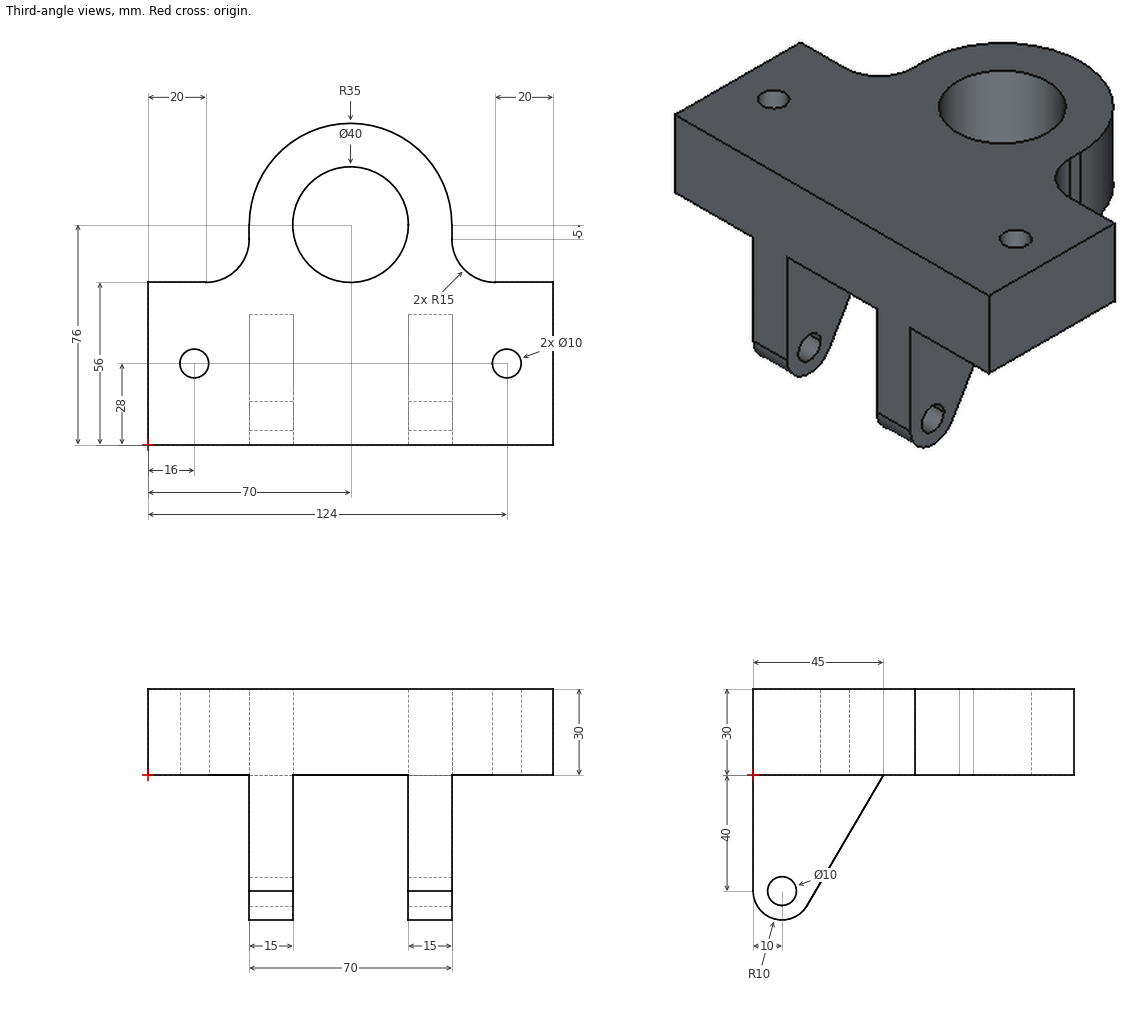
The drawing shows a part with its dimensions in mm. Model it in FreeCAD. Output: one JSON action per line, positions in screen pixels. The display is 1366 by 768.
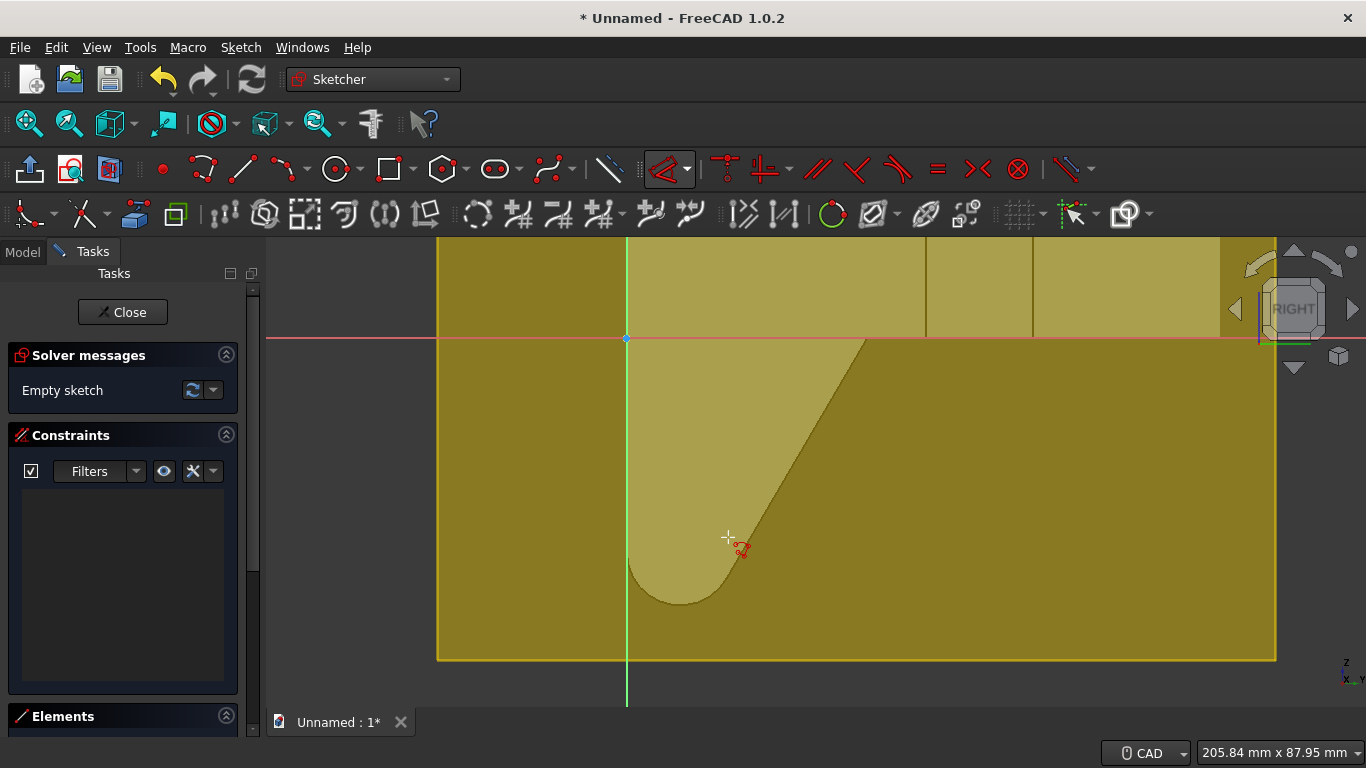
{"action": "left_click", "coordinate": [726, 579]}
{"action": "left_click", "coordinate": [867, 338]}
{"action": "left_click", "coordinate": [627, 338]}
{"action": "left_click", "coordinate": [636, 552]}
{"action": "right_click", "coordinate": [636, 552]}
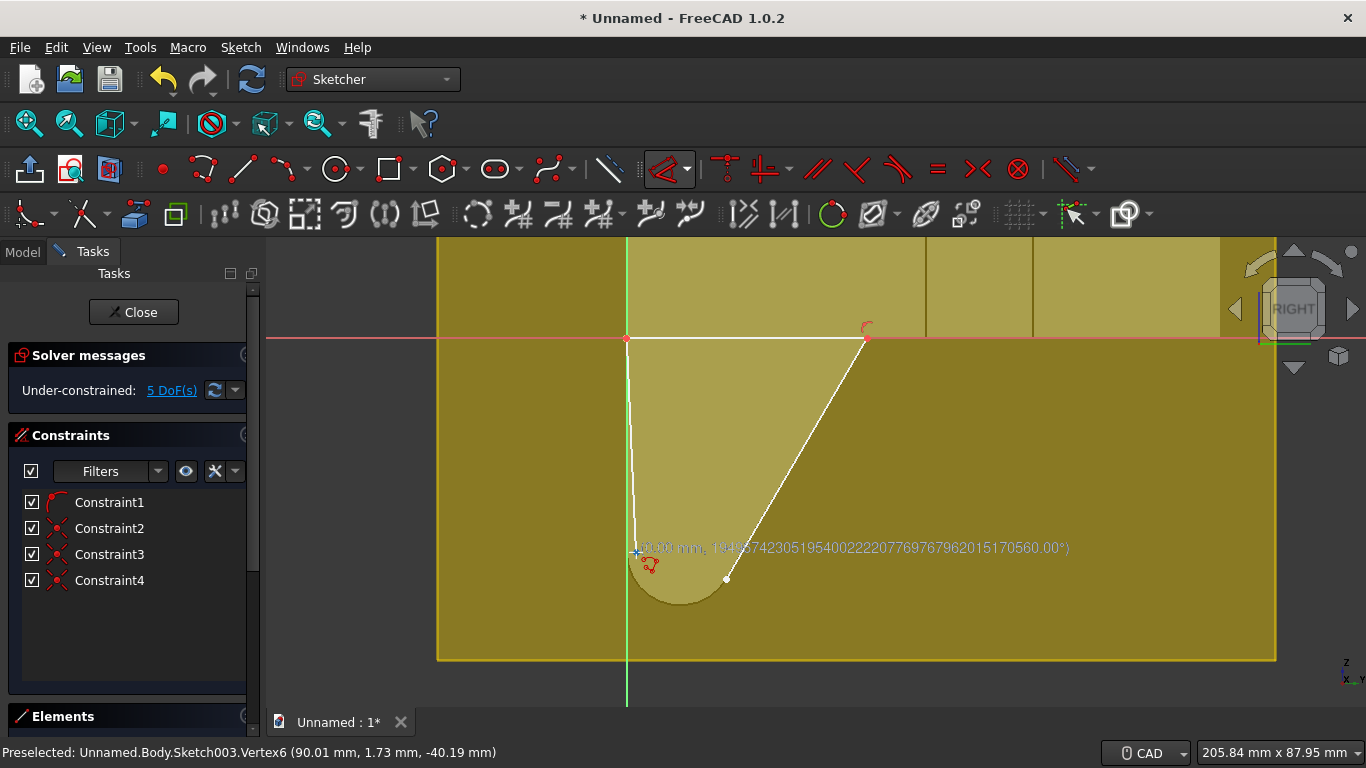
{"action": "left_click", "coordinate": [284, 170]}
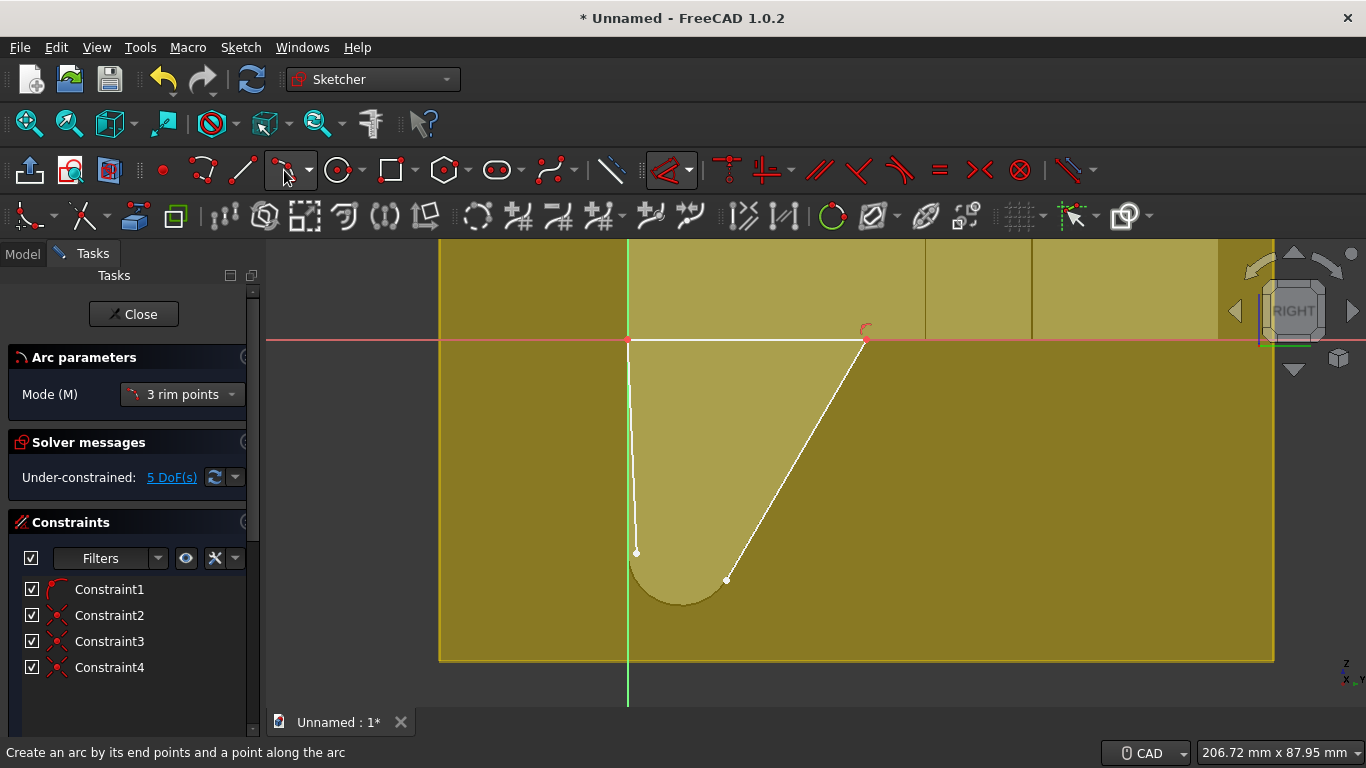
{"action": "left_click", "coordinate": [637, 554]}
{"action": "left_click", "coordinate": [726, 581]}
{"action": "left_click", "coordinate": [667, 604]}
{"action": "key", "text": "Escape"}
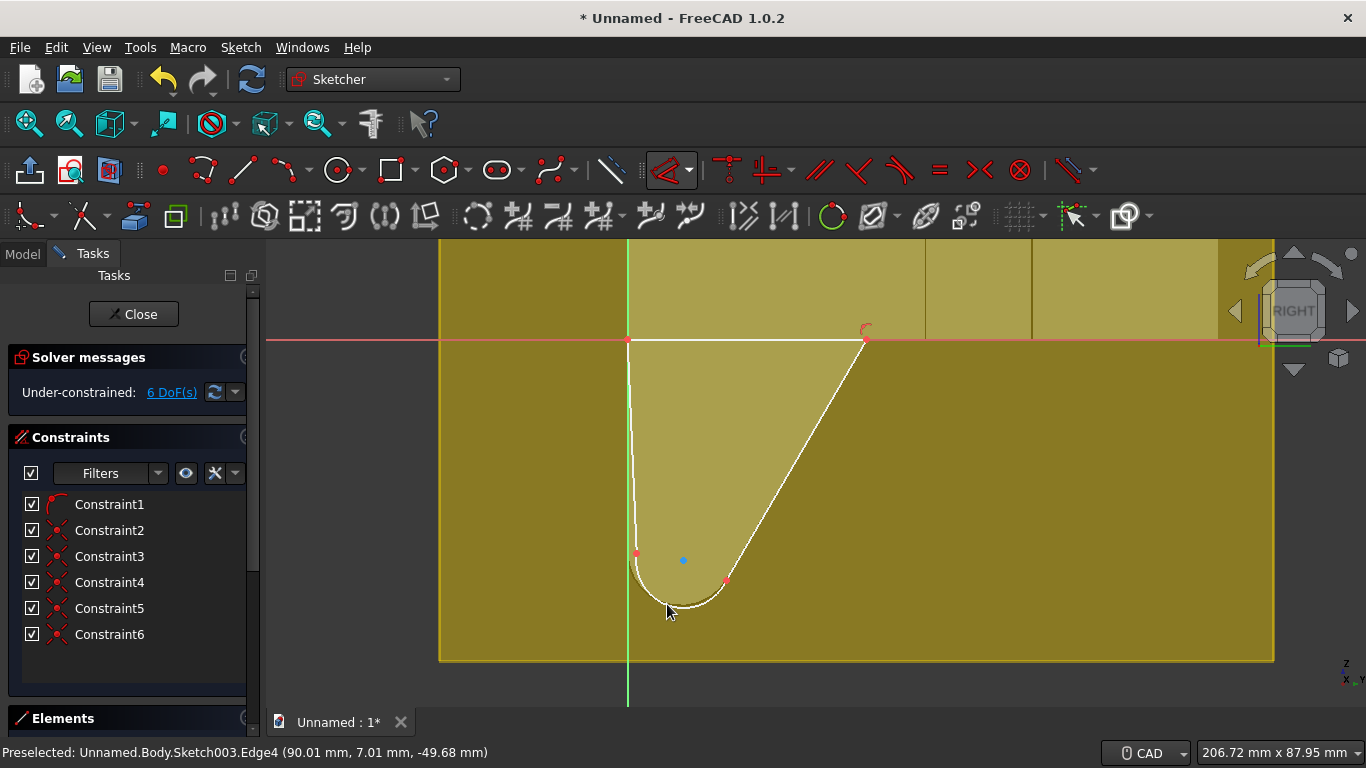
{"action": "left_click", "coordinate": [769, 508]}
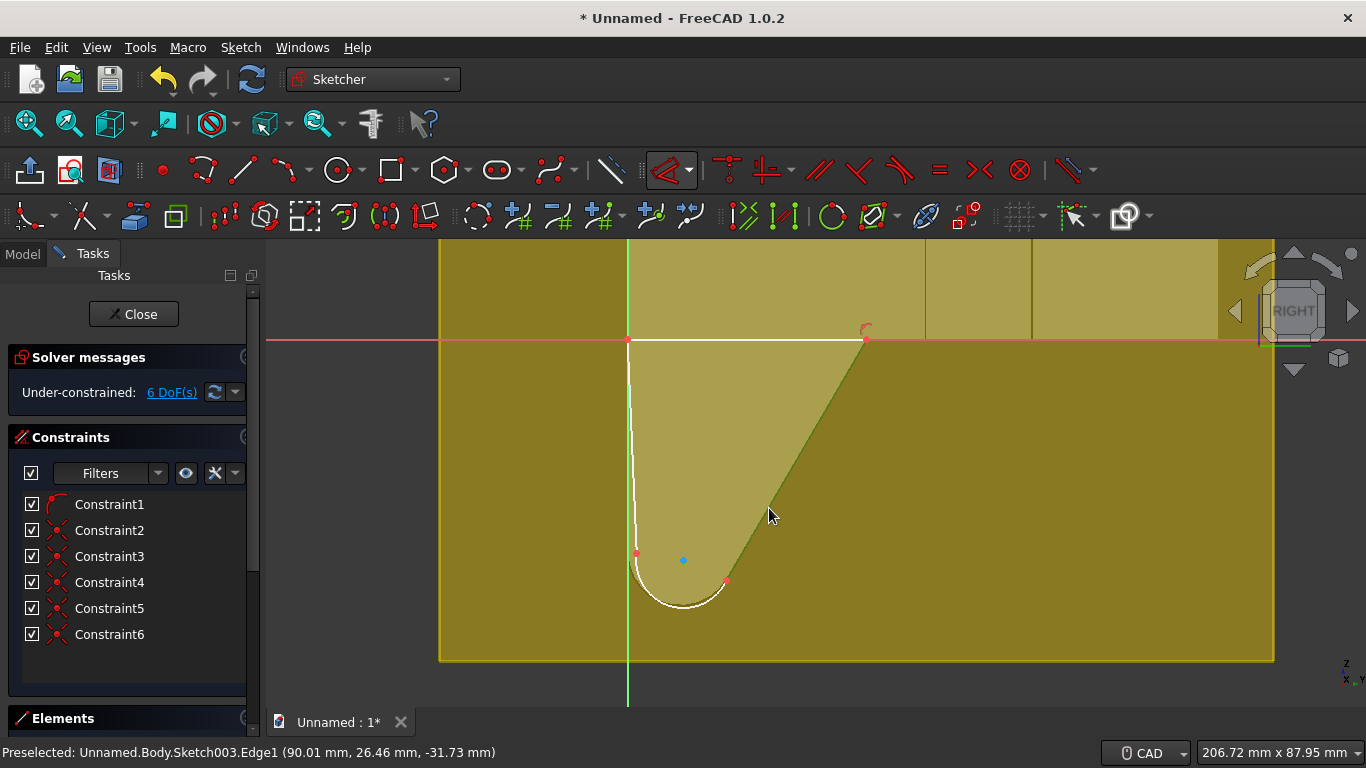
{"action": "left_click", "coordinate": [648, 591]}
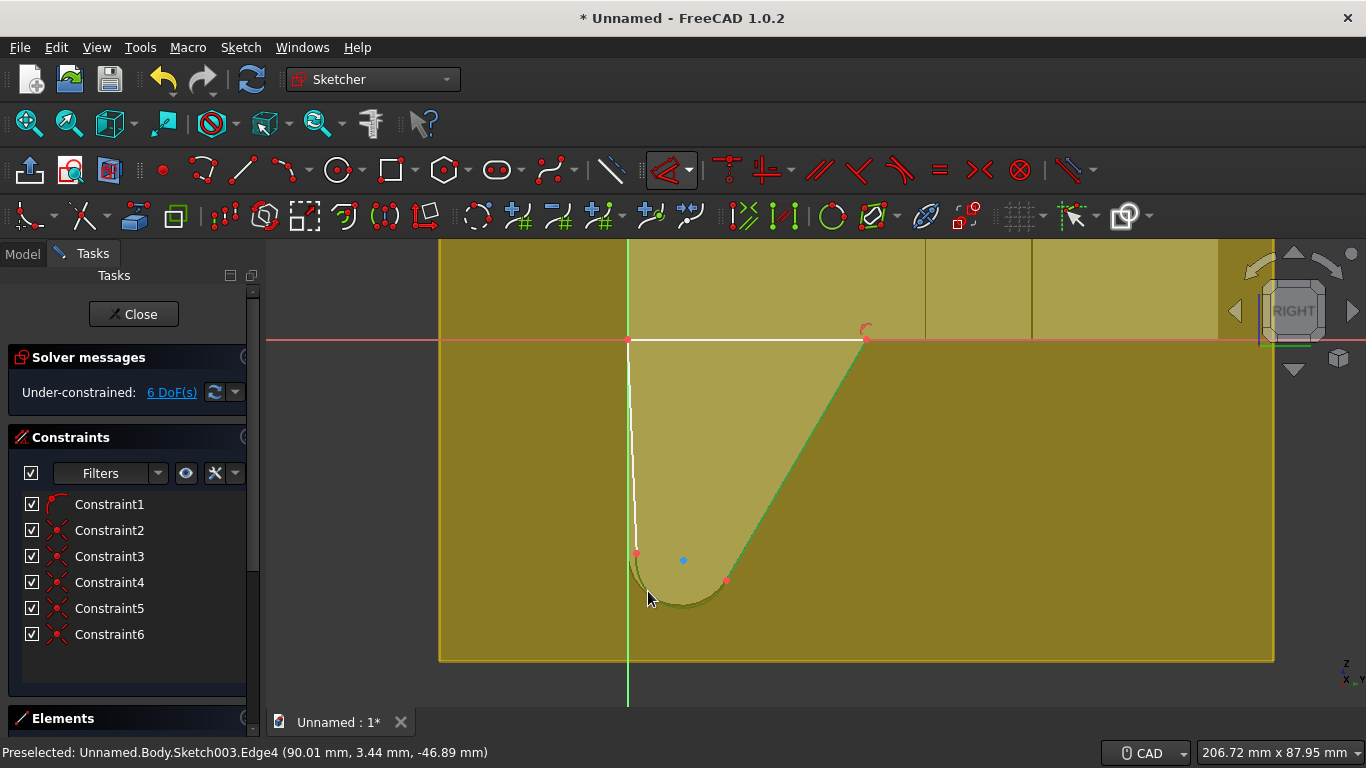
{"action": "left_click", "coordinate": [900, 170]}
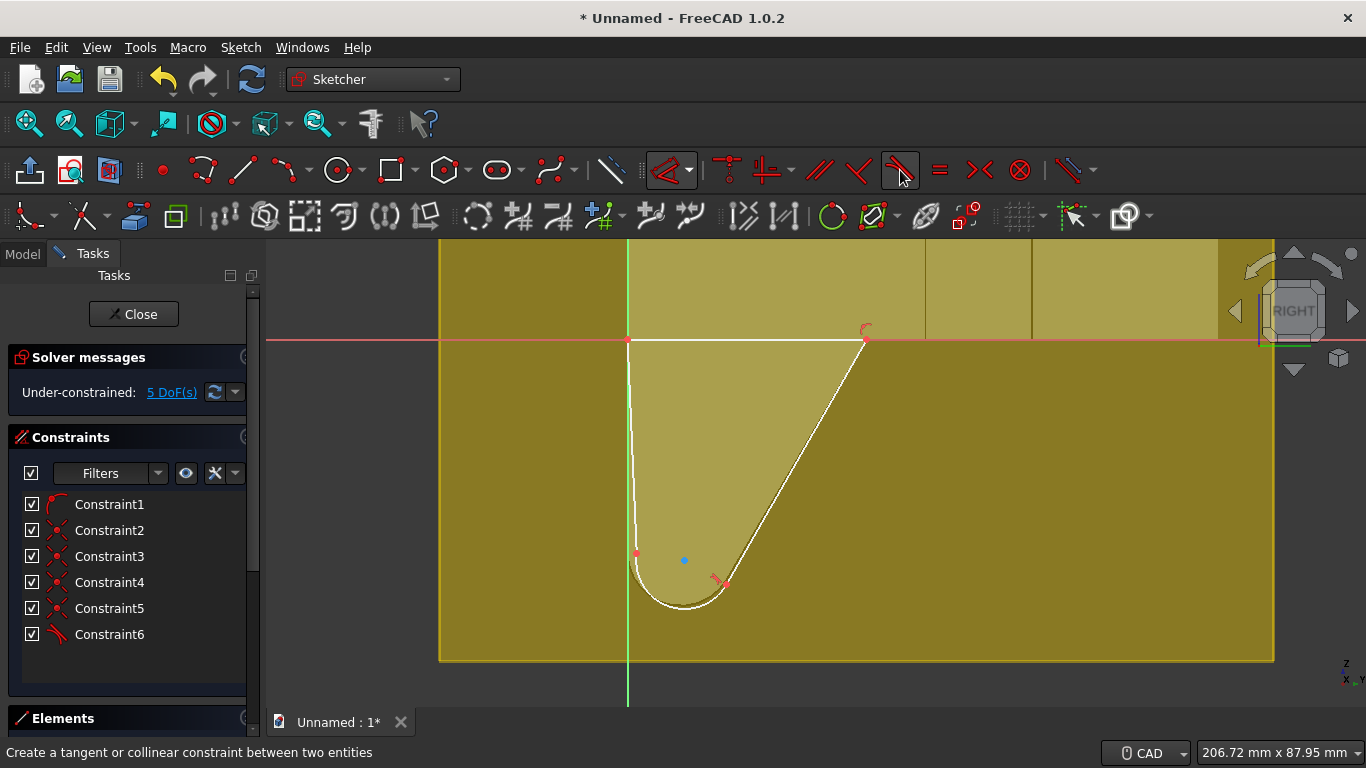
{"action": "left_click", "coordinate": [630, 404]}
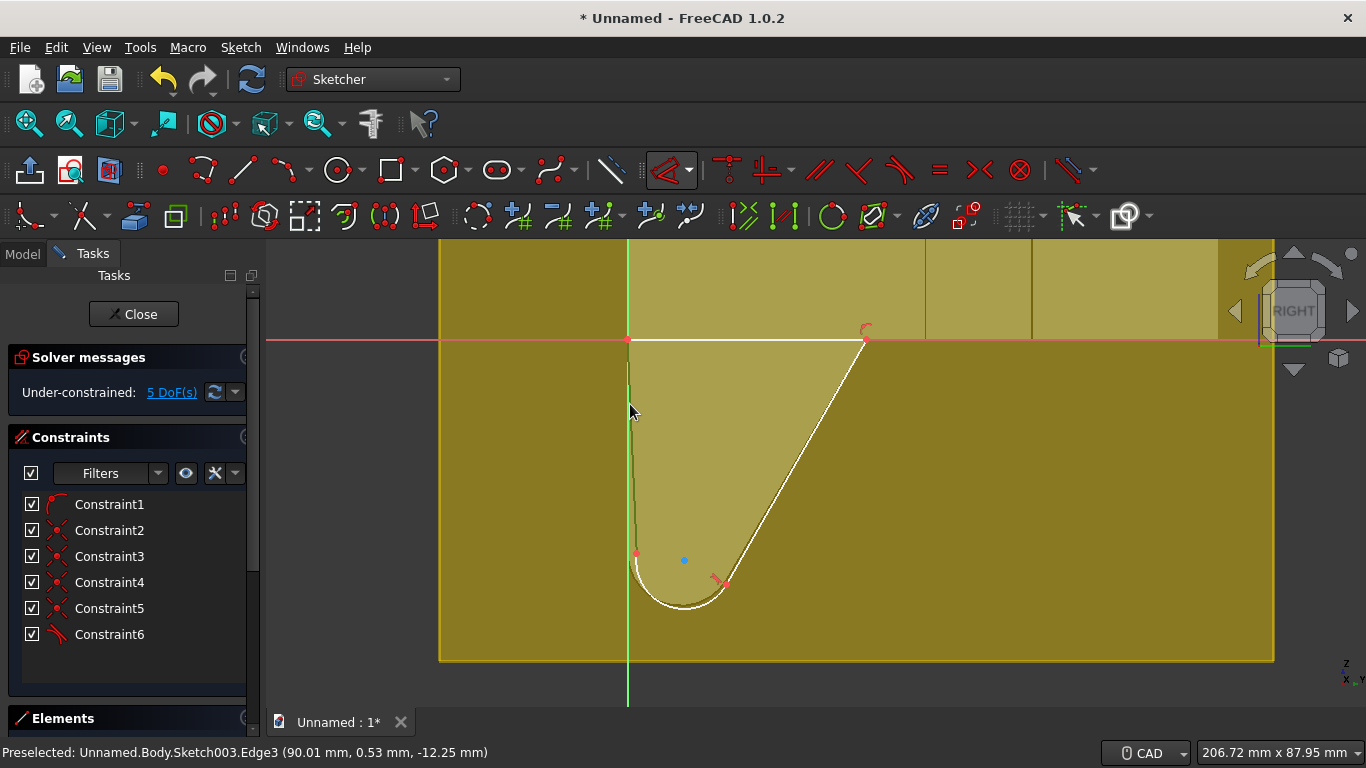
{"action": "left_click", "coordinate": [647, 591]}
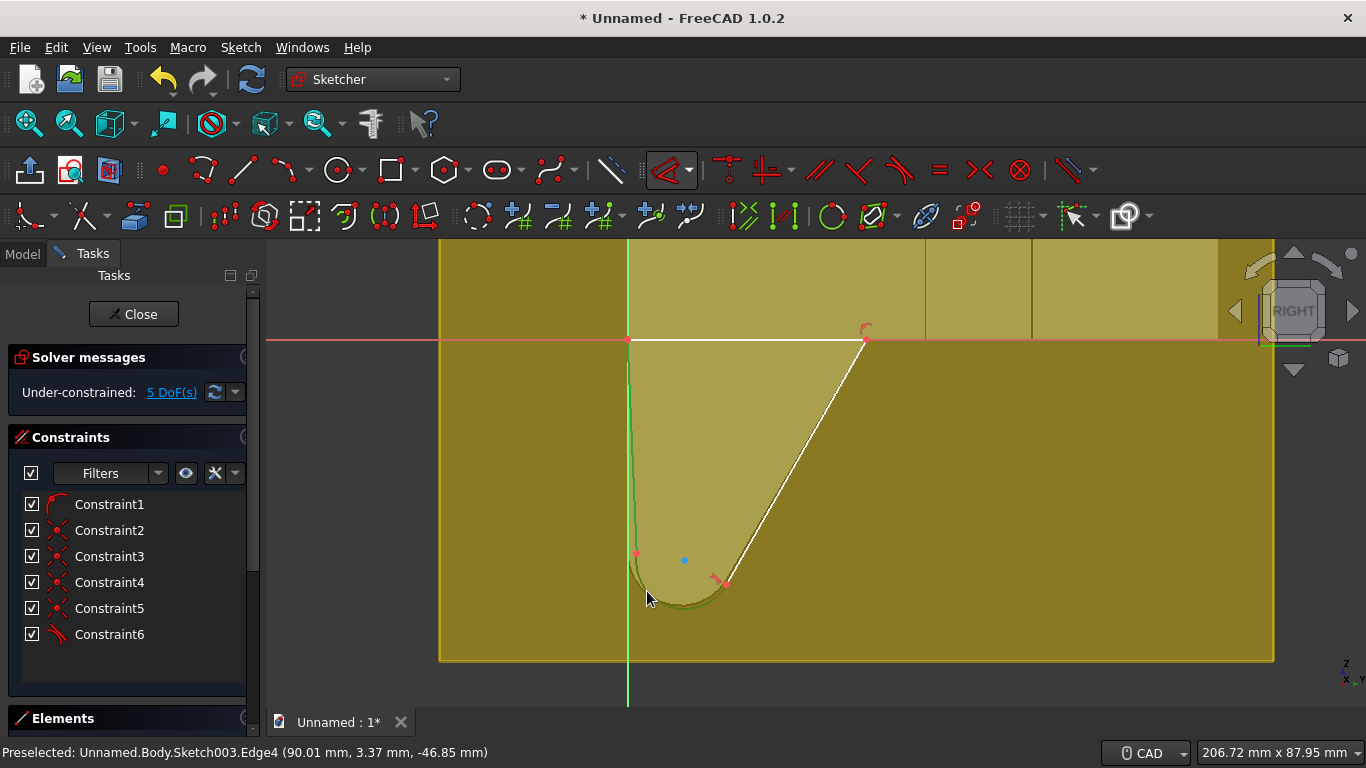
{"action": "left_click", "coordinate": [900, 170]}